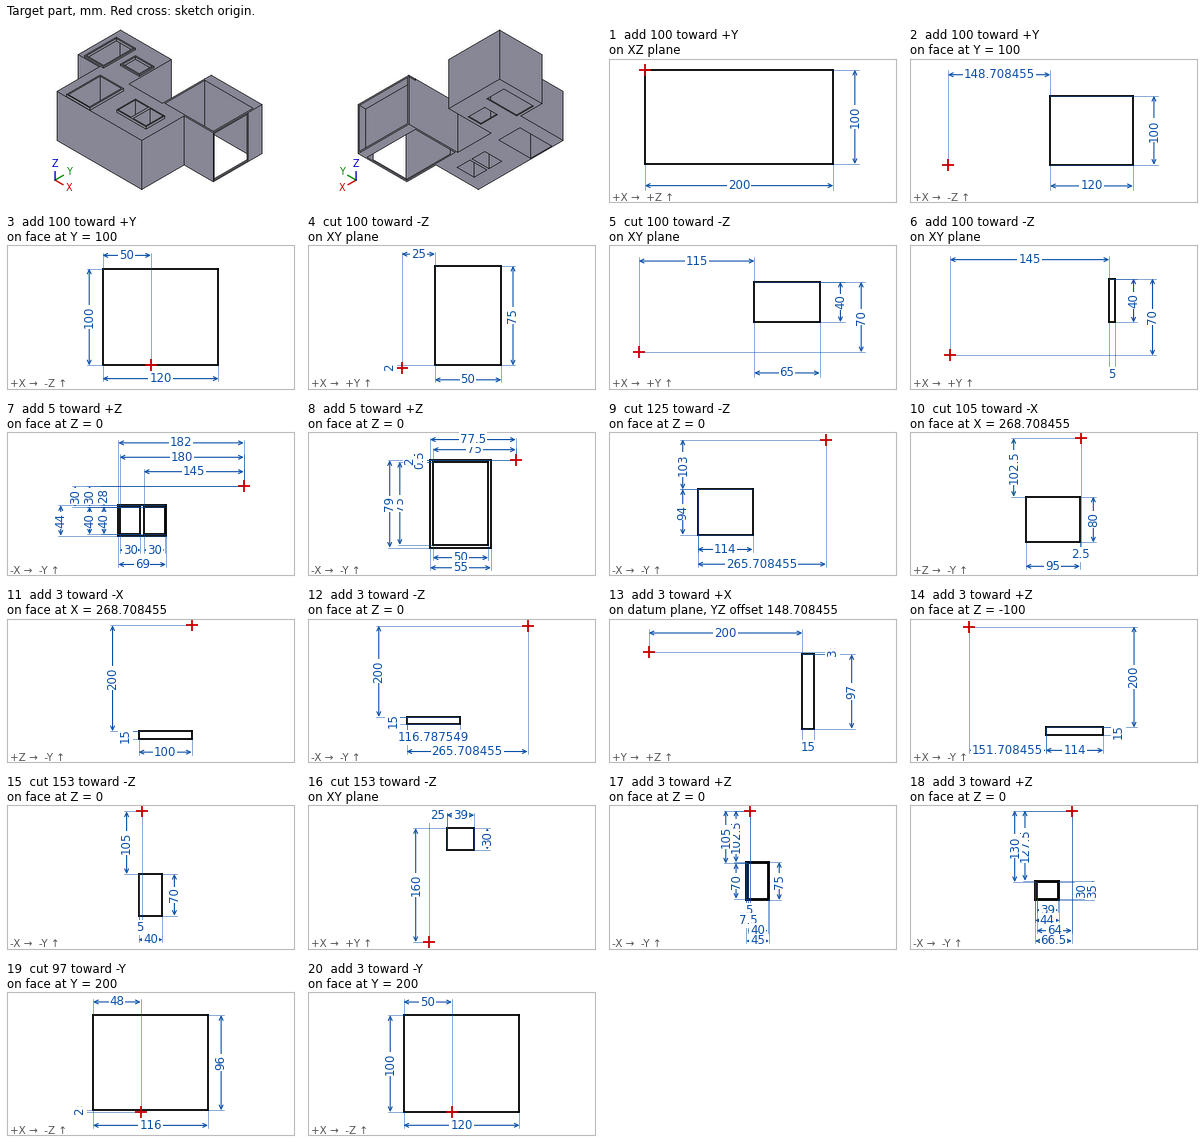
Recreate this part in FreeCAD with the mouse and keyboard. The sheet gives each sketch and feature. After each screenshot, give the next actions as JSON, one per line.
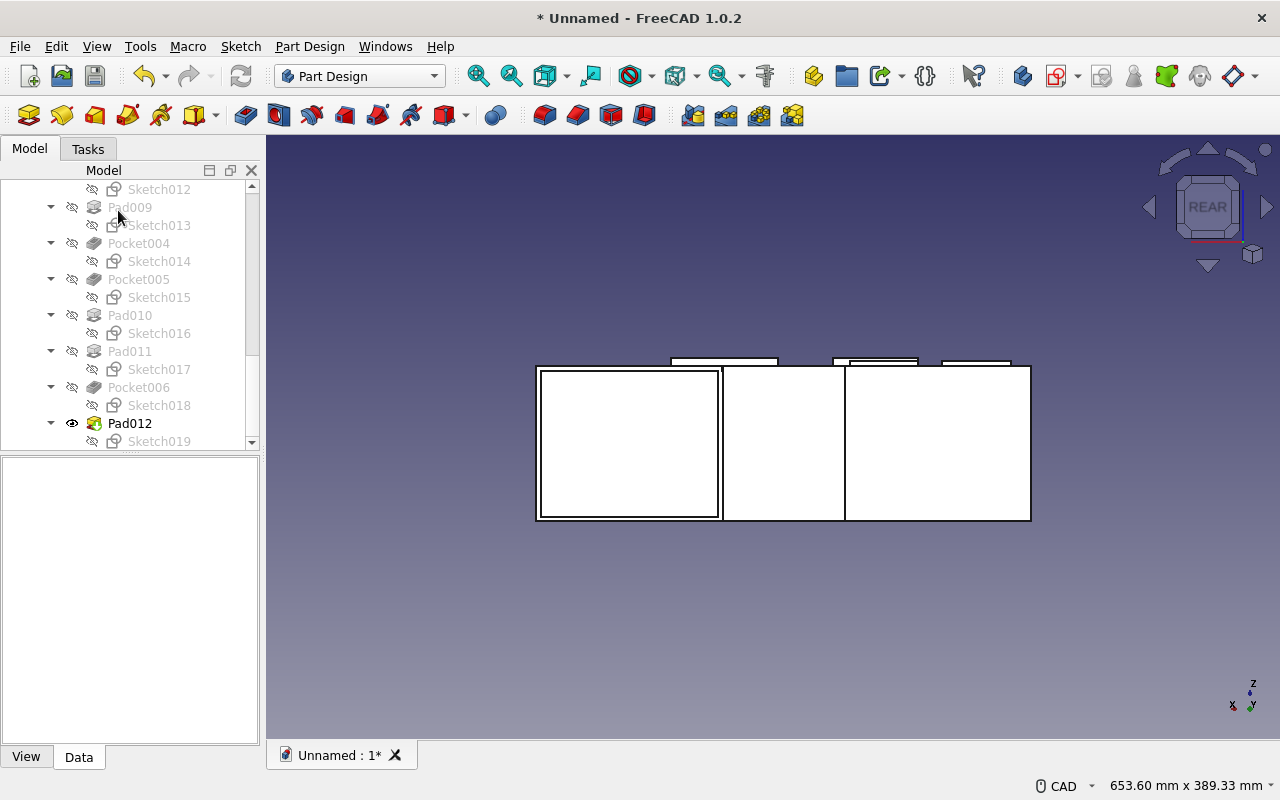
{"action": "key", "text": "0"}